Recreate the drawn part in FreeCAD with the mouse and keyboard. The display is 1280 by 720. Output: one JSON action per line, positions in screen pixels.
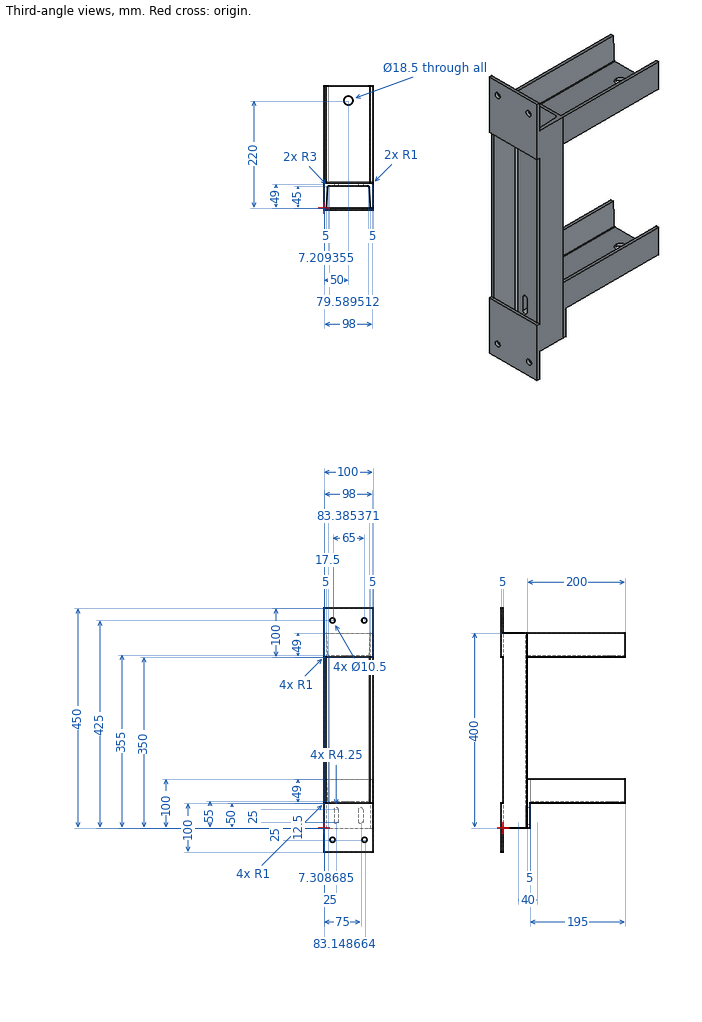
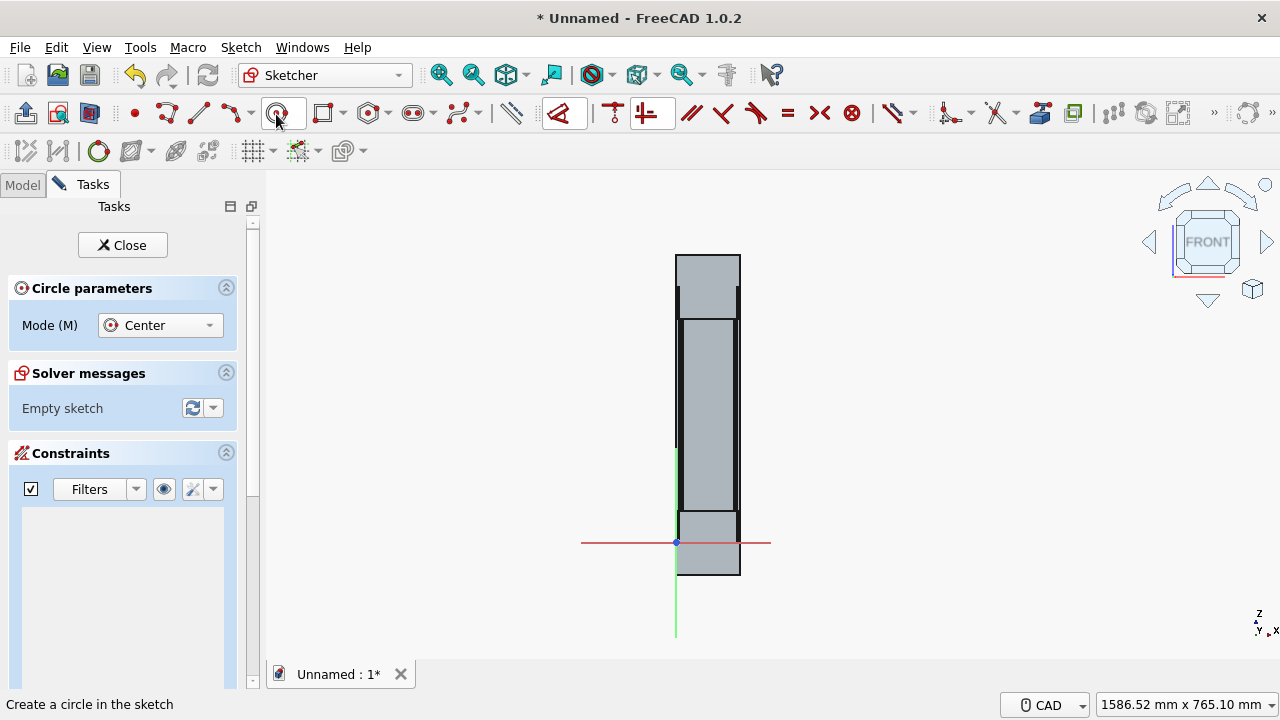
{"action": "scroll", "coordinate": [687, 271], "scroll_direction": "up", "scroll_amount": 10}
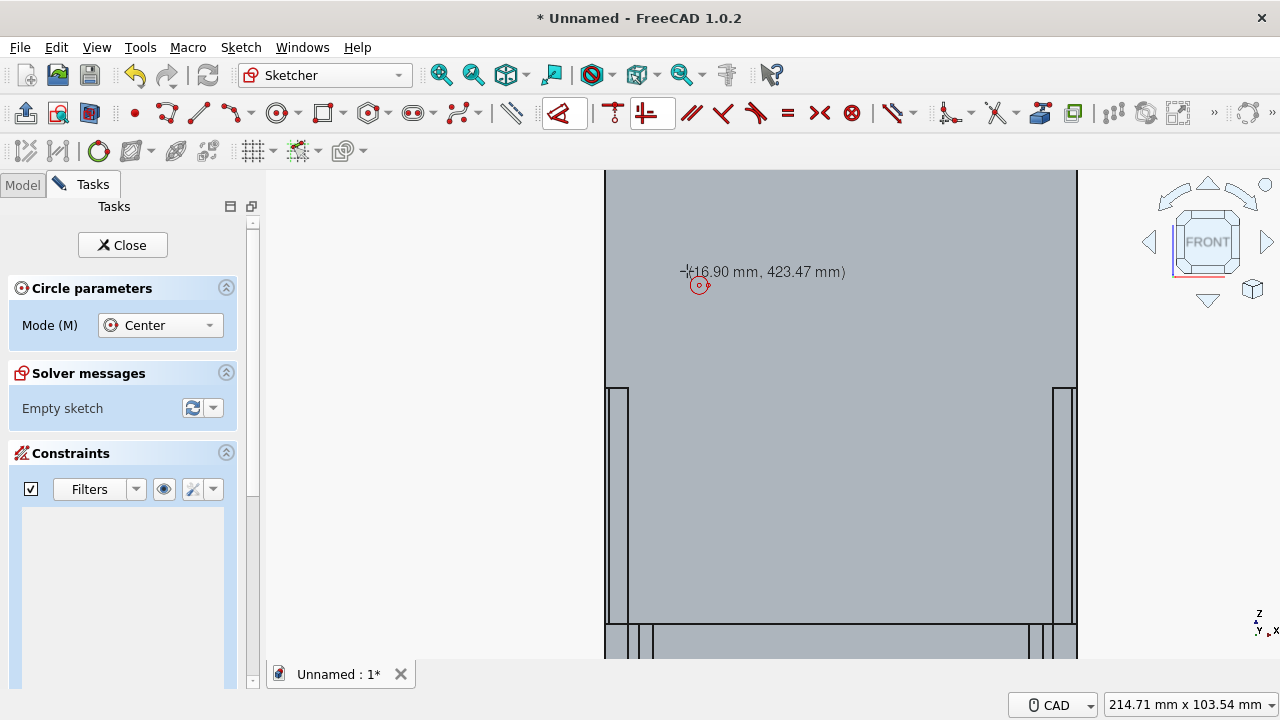
{"action": "scroll", "coordinate": [687, 271], "scroll_direction": "down", "scroll_amount": 10}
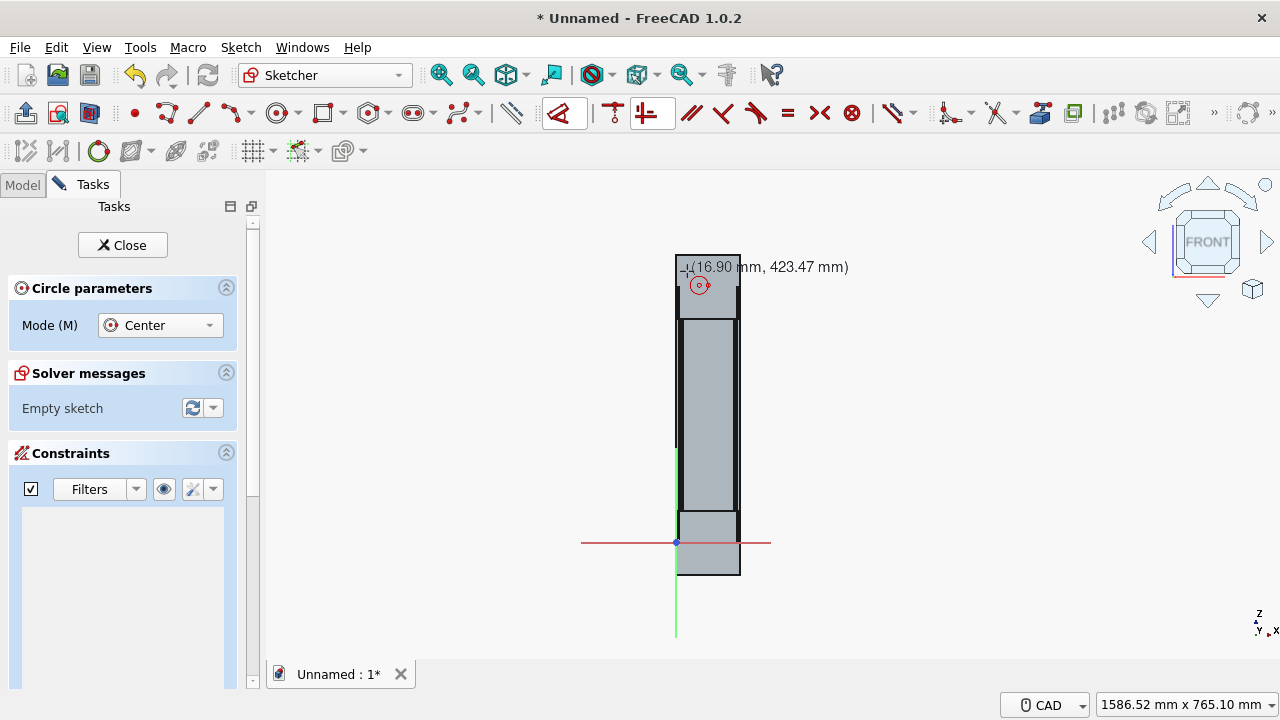
{"action": "scroll", "coordinate": [687, 271], "scroll_direction": "up", "scroll_amount": 2}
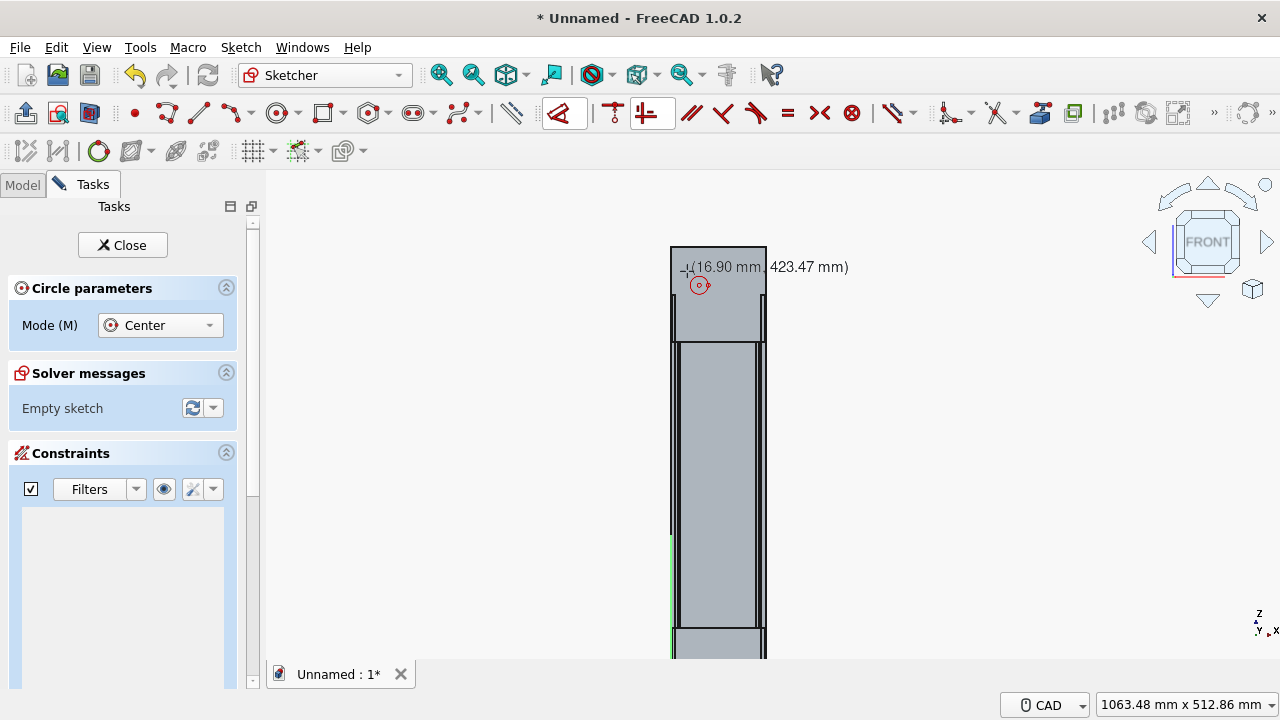
{"action": "left_click", "coordinate": [687, 271]}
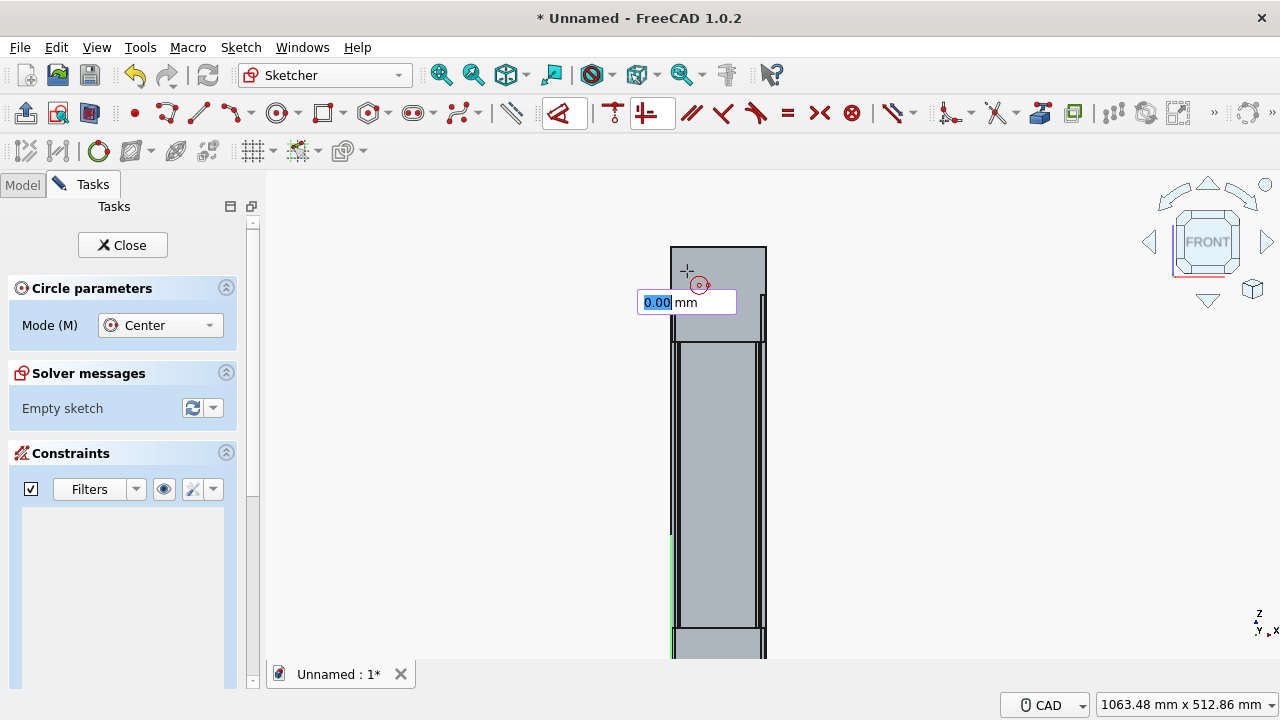
{"action": "scroll", "coordinate": [691, 267], "scroll_direction": "up", "scroll_amount": 6}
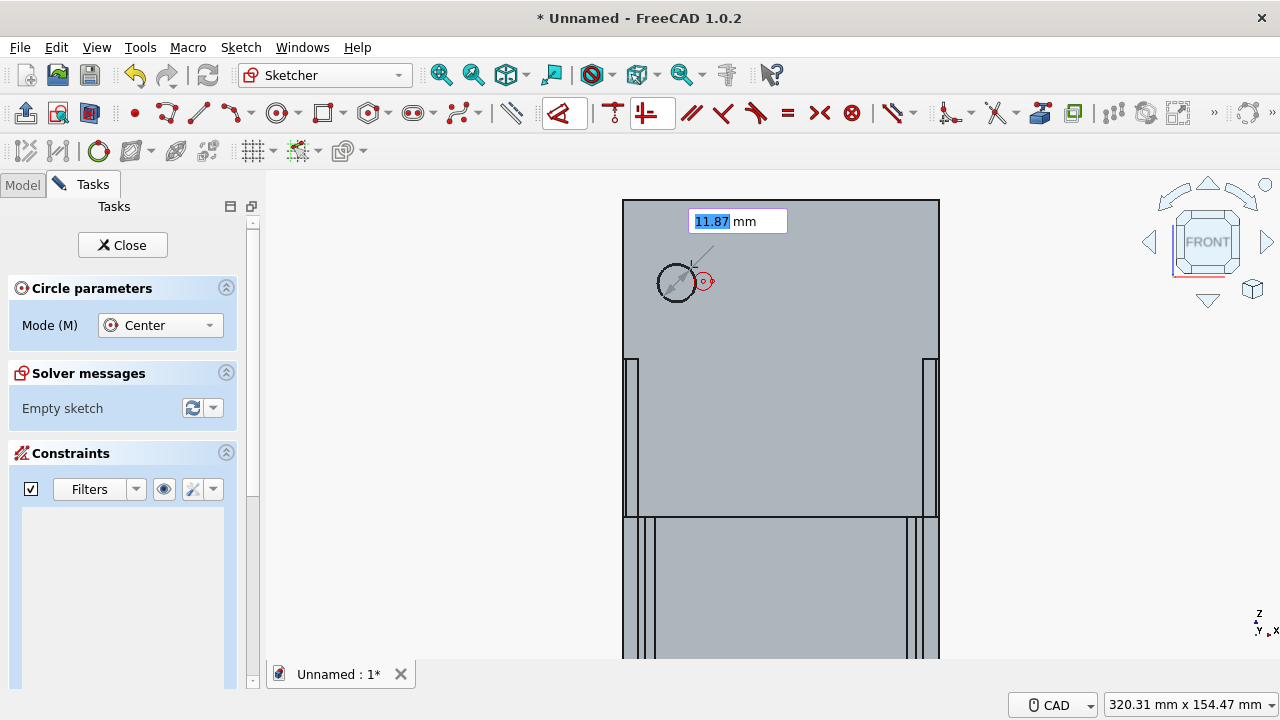
{"action": "left_click", "coordinate": [690, 268]}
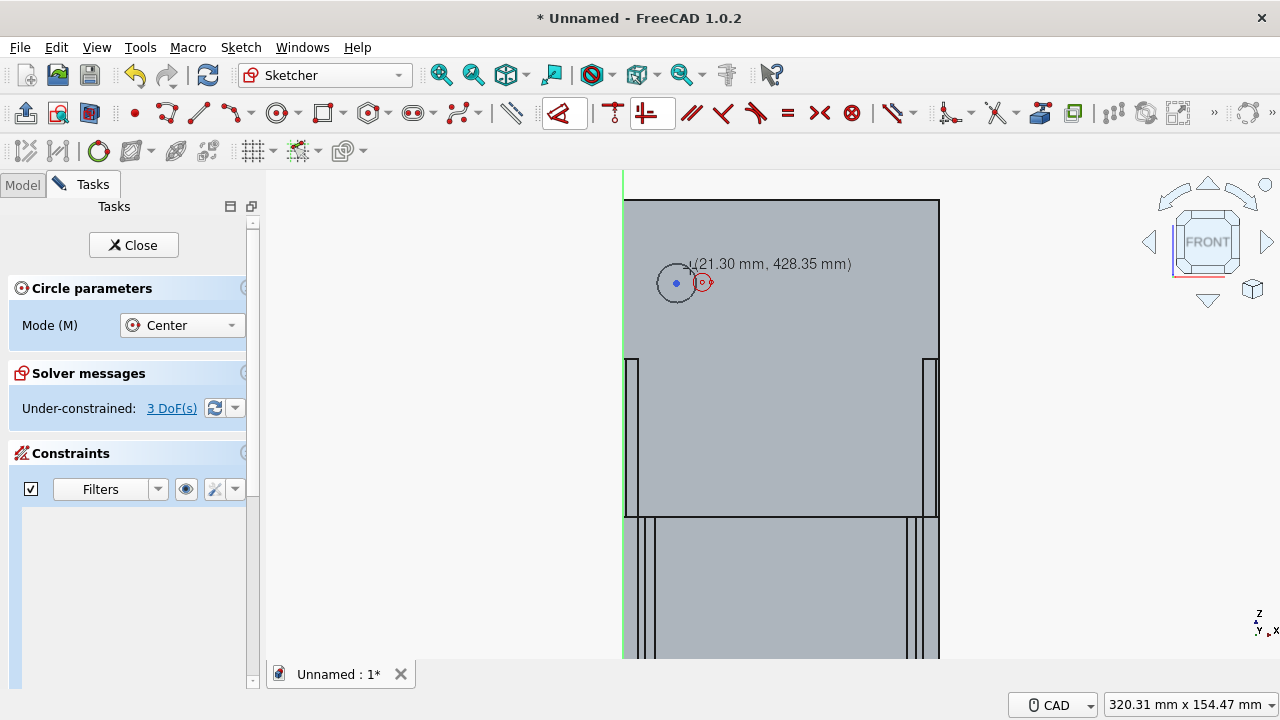
{"action": "scroll", "coordinate": [884, 280], "scroll_direction": "up", "scroll_amount": 2}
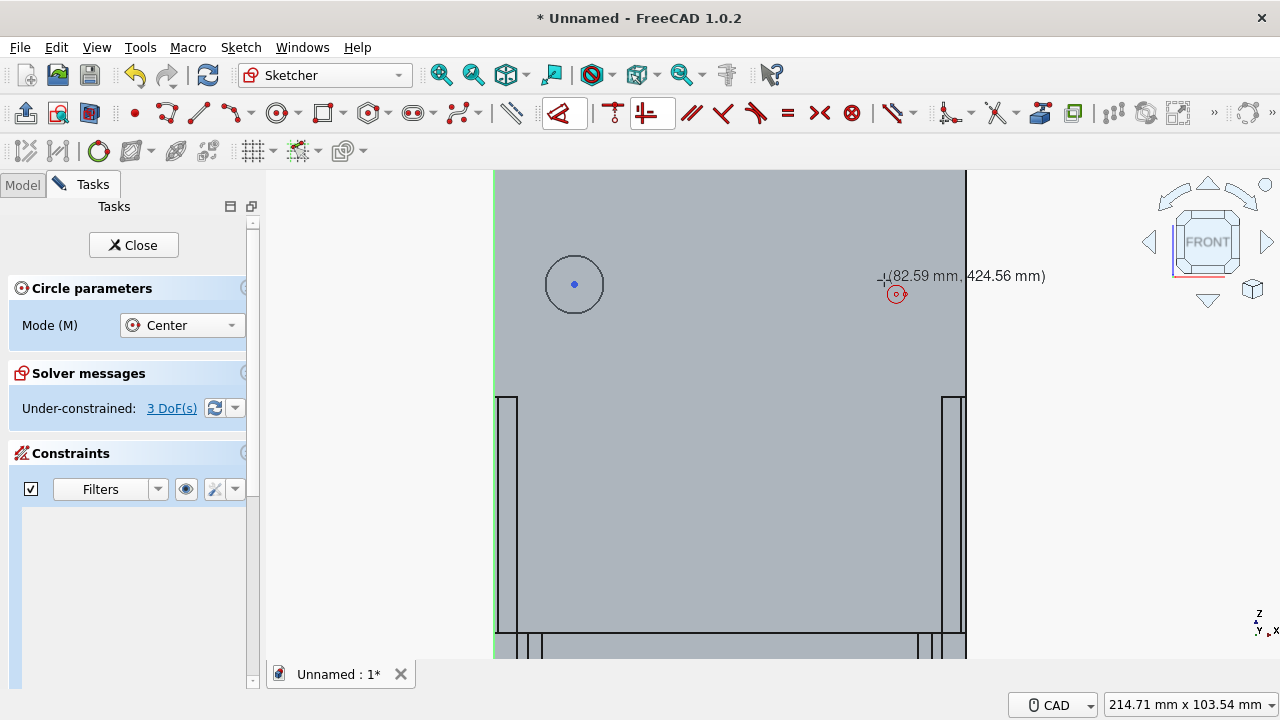
{"action": "scroll", "coordinate": [705, 269], "scroll_direction": "down", "scroll_amount": 10}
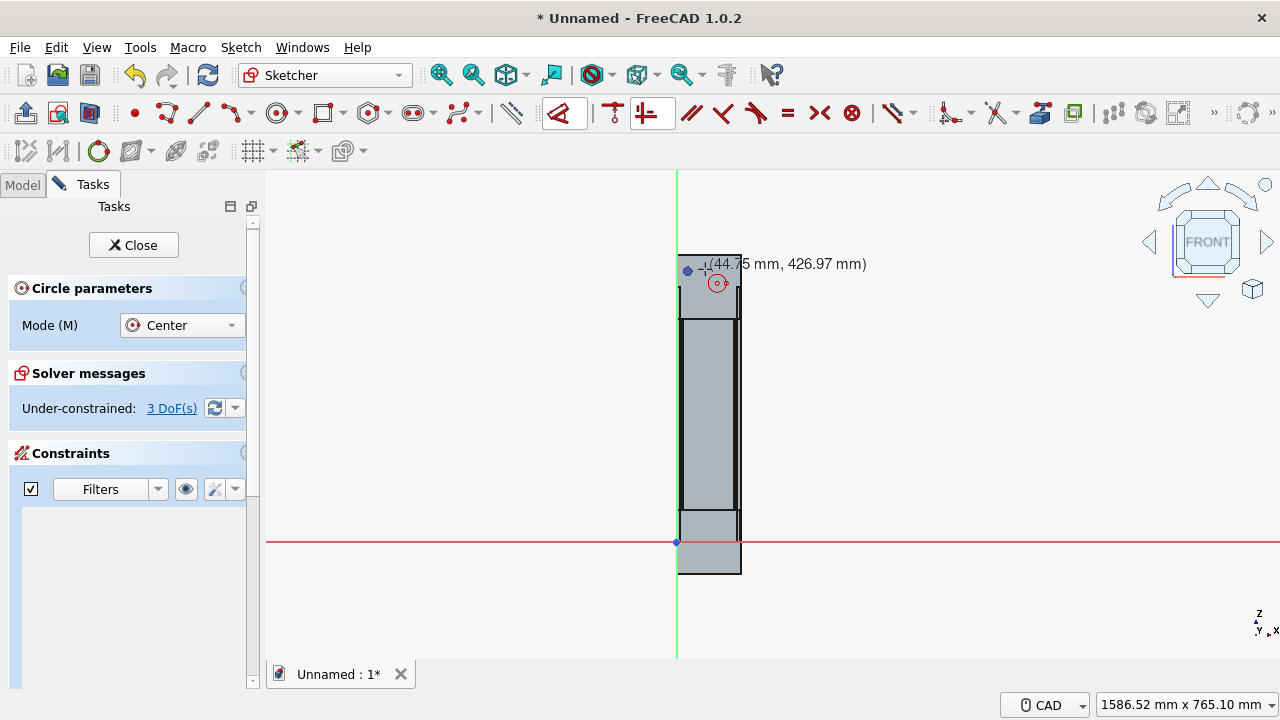
{"action": "left_click", "coordinate": [730, 271]}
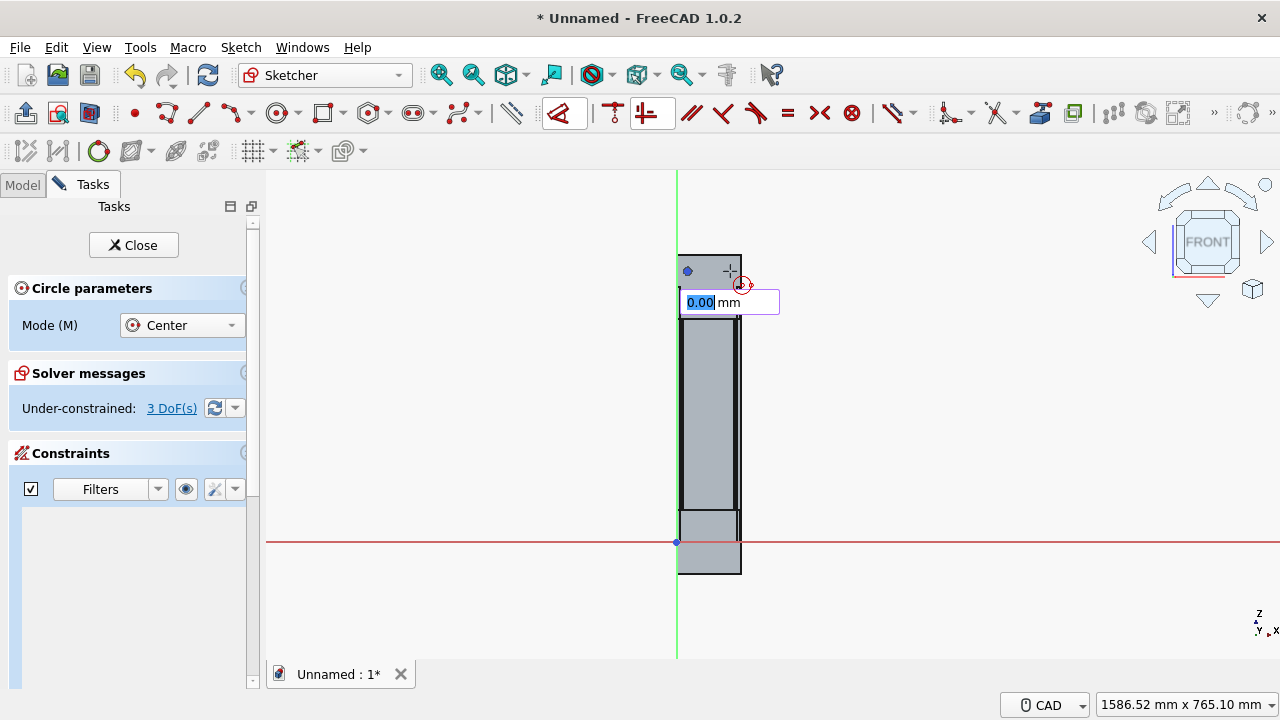
{"action": "scroll", "coordinate": [732, 268], "scroll_direction": "up", "scroll_amount": 8}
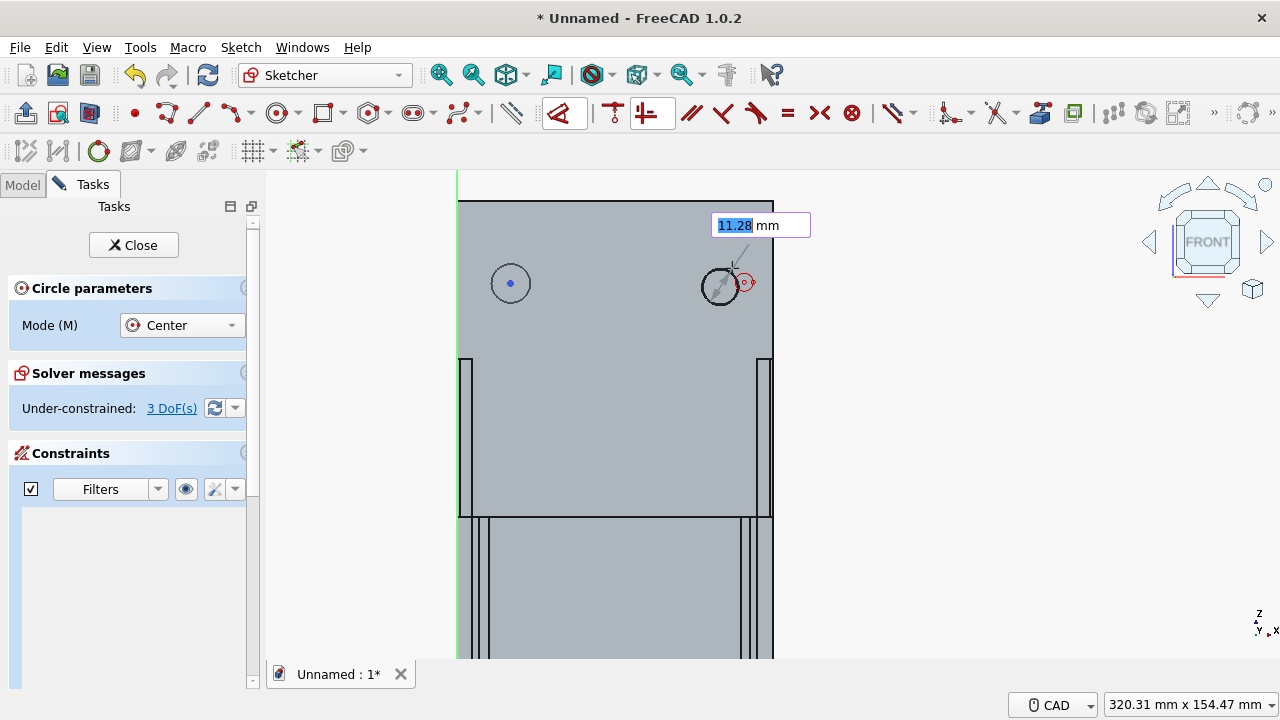
{"action": "left_click", "coordinate": [730, 268]}